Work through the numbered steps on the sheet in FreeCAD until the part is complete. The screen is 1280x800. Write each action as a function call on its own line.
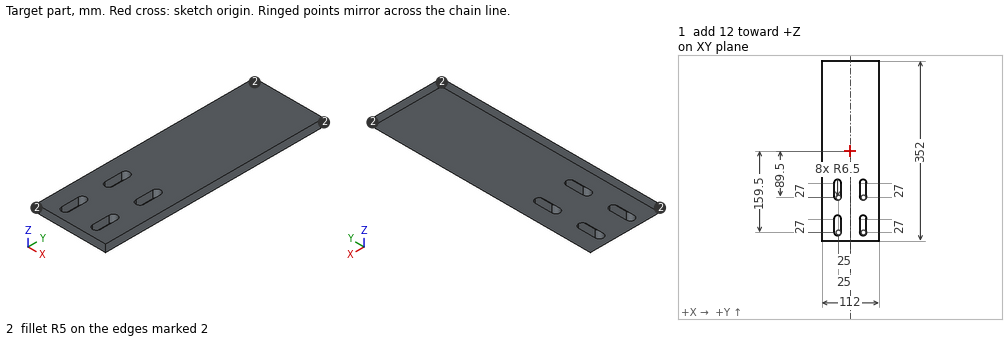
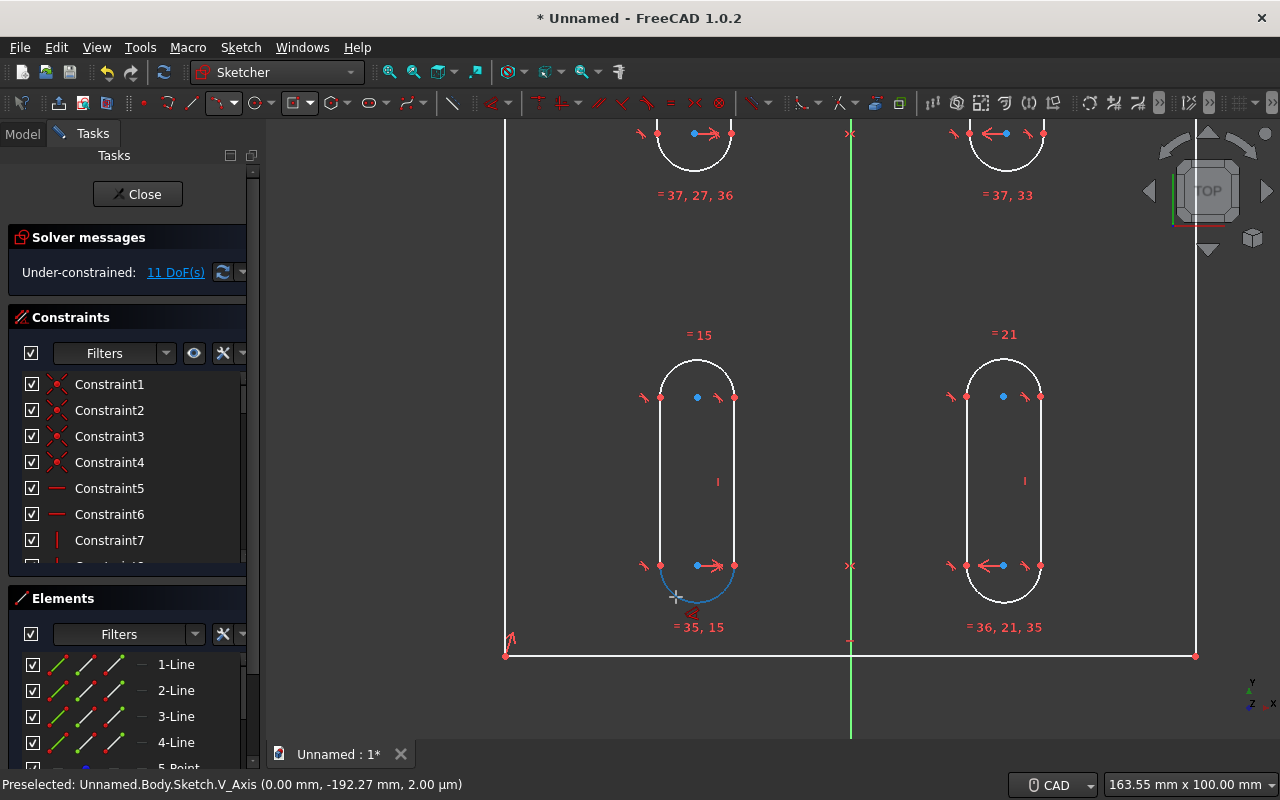
click(675, 596)
click(656, 622)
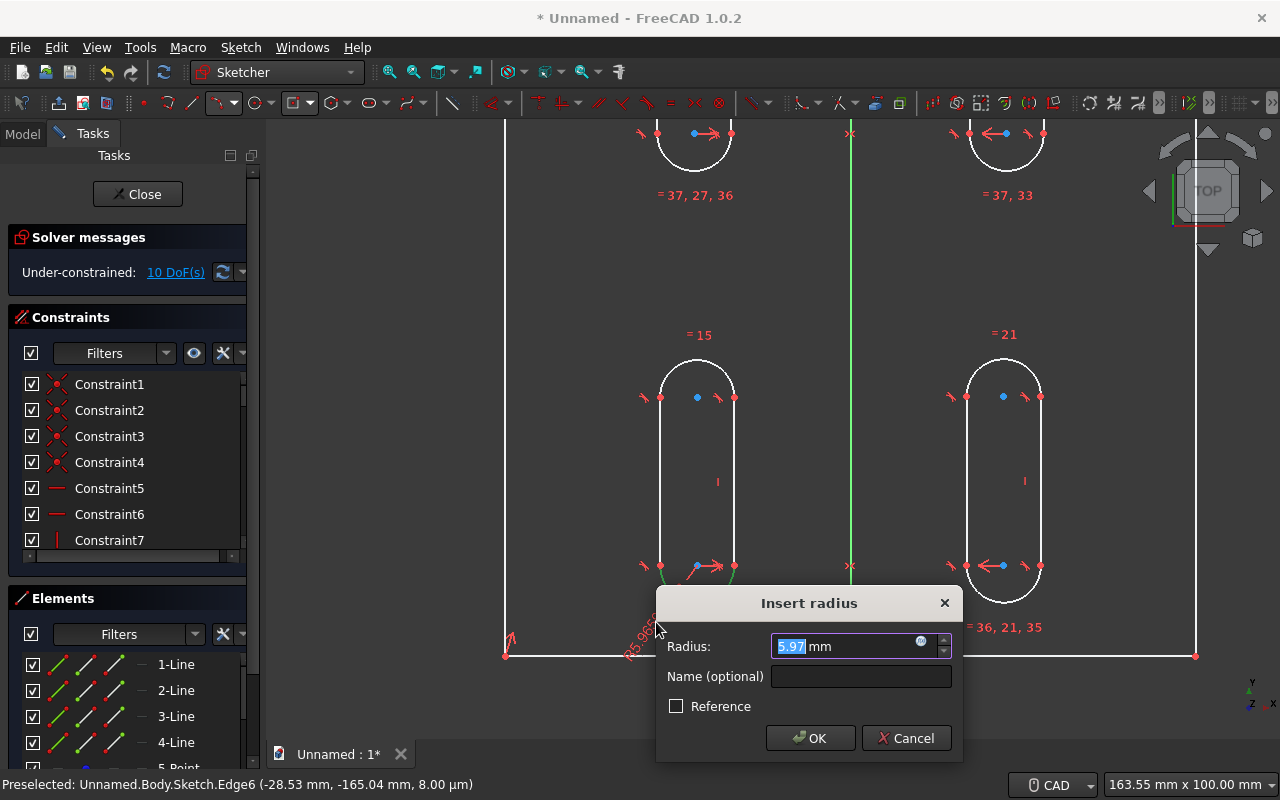
text(6.5)
key(Return)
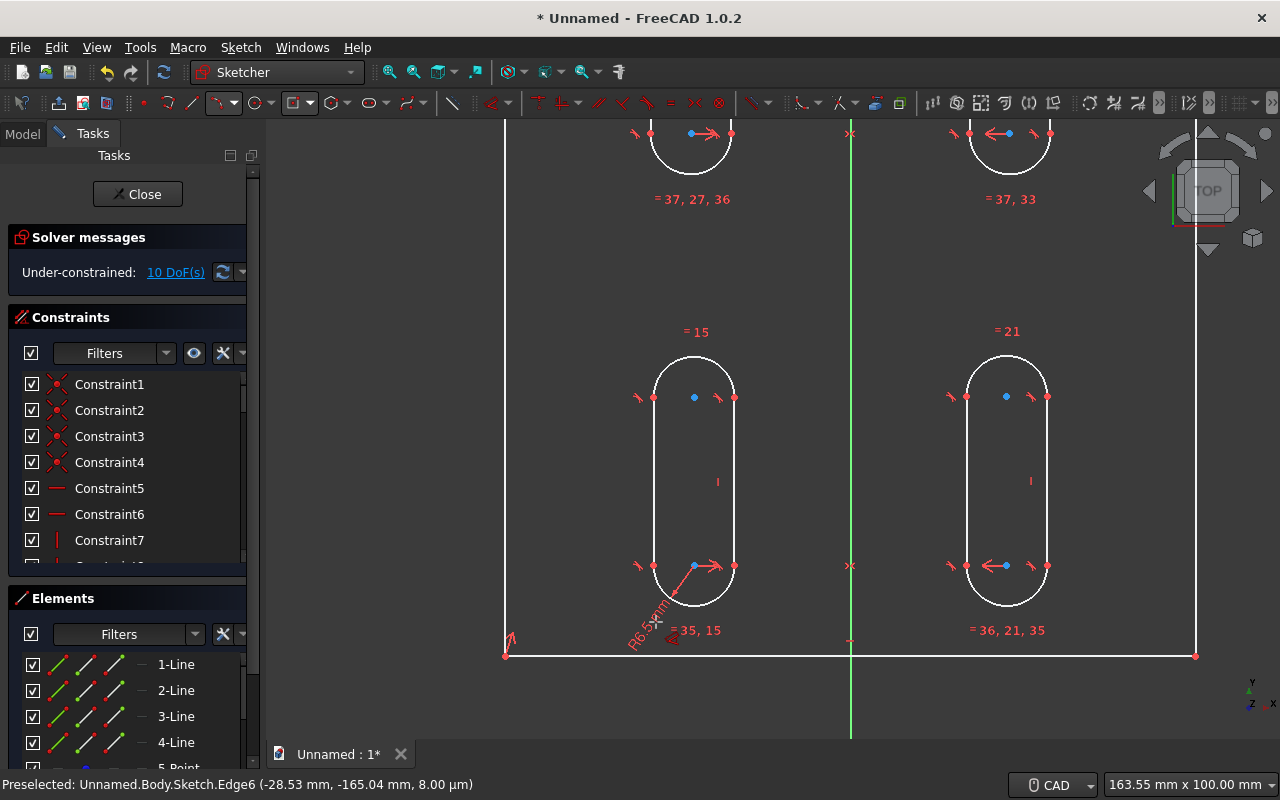
scroll(676, 599, down, 9)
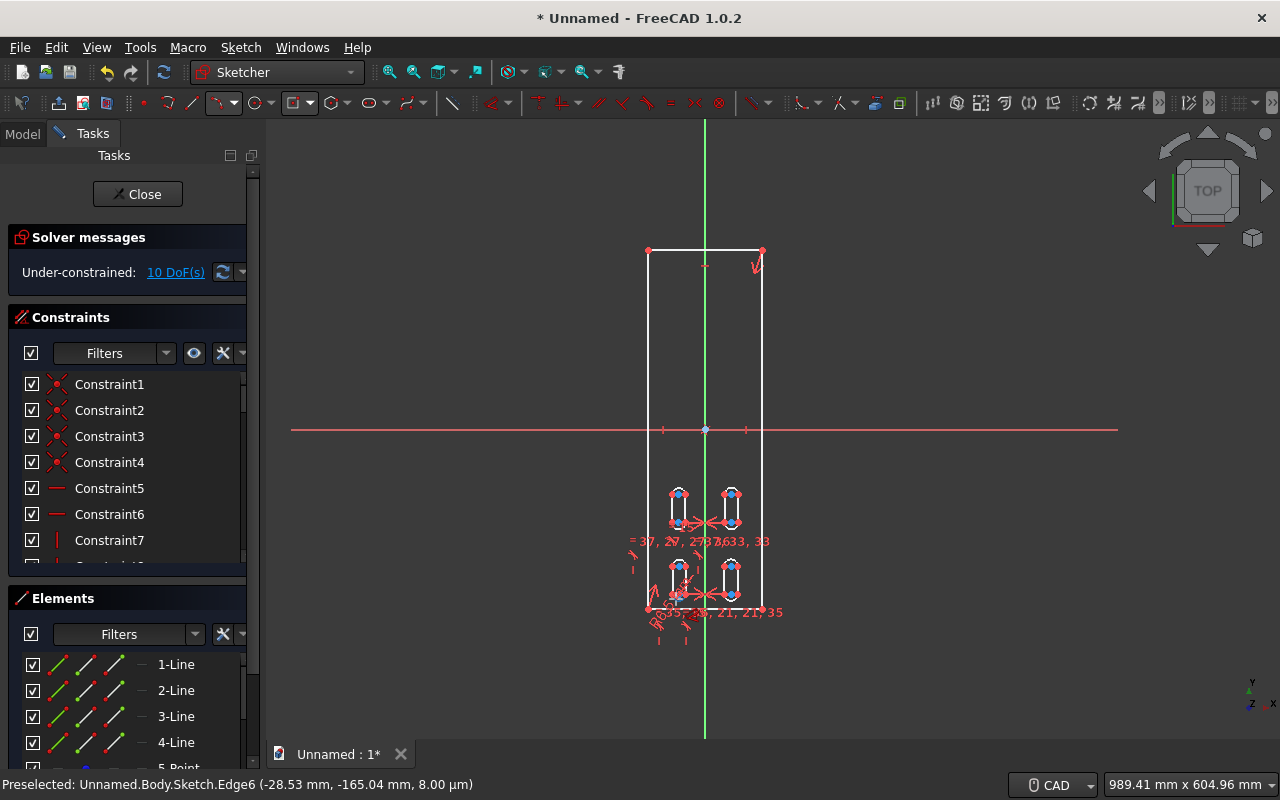
scroll(673, 586, up, 3)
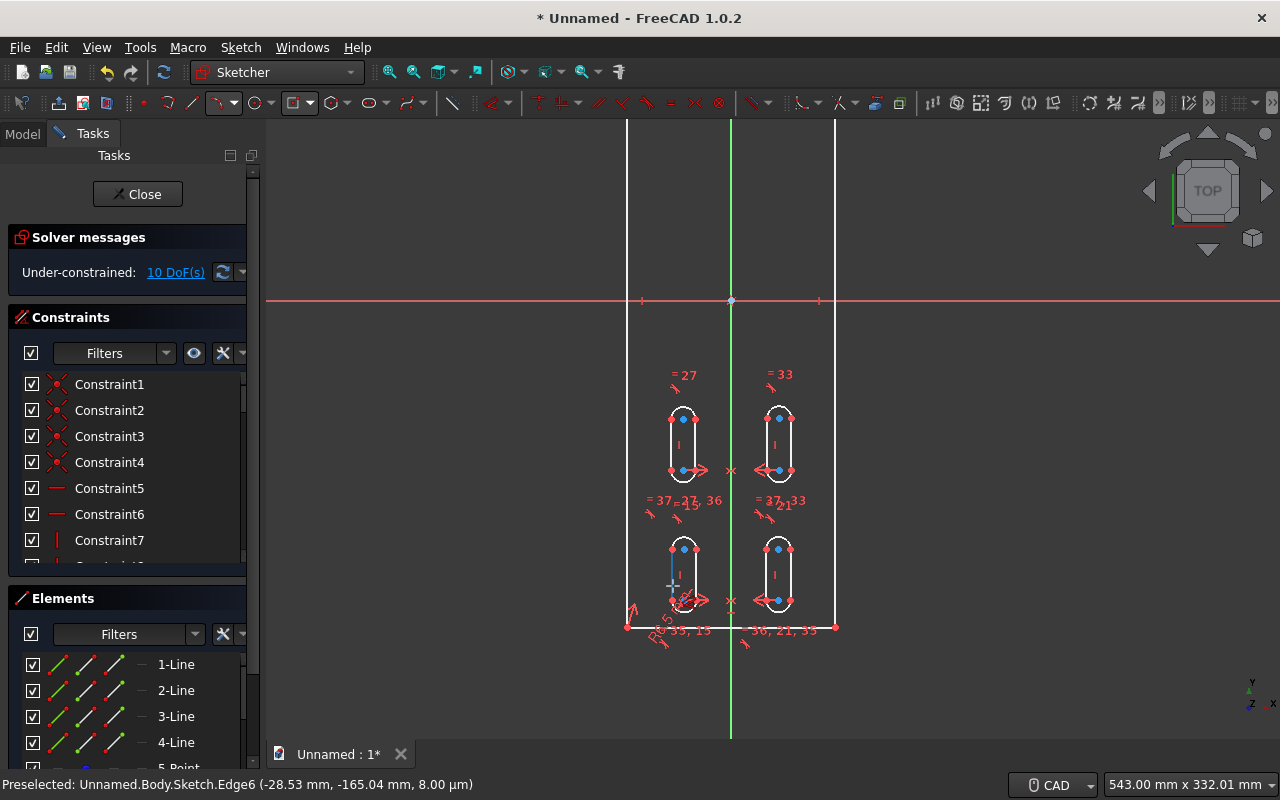
click(672, 585)
click(614, 575)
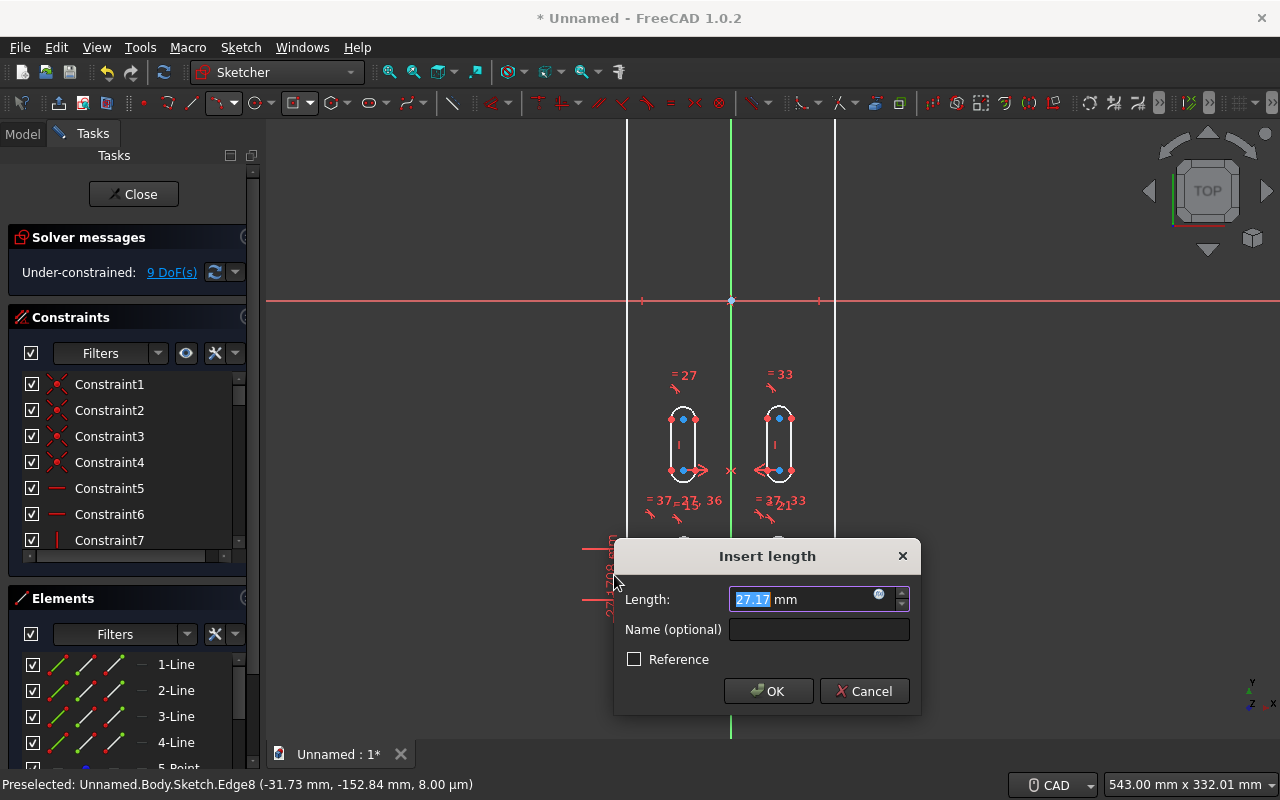
text(27)
key(Return)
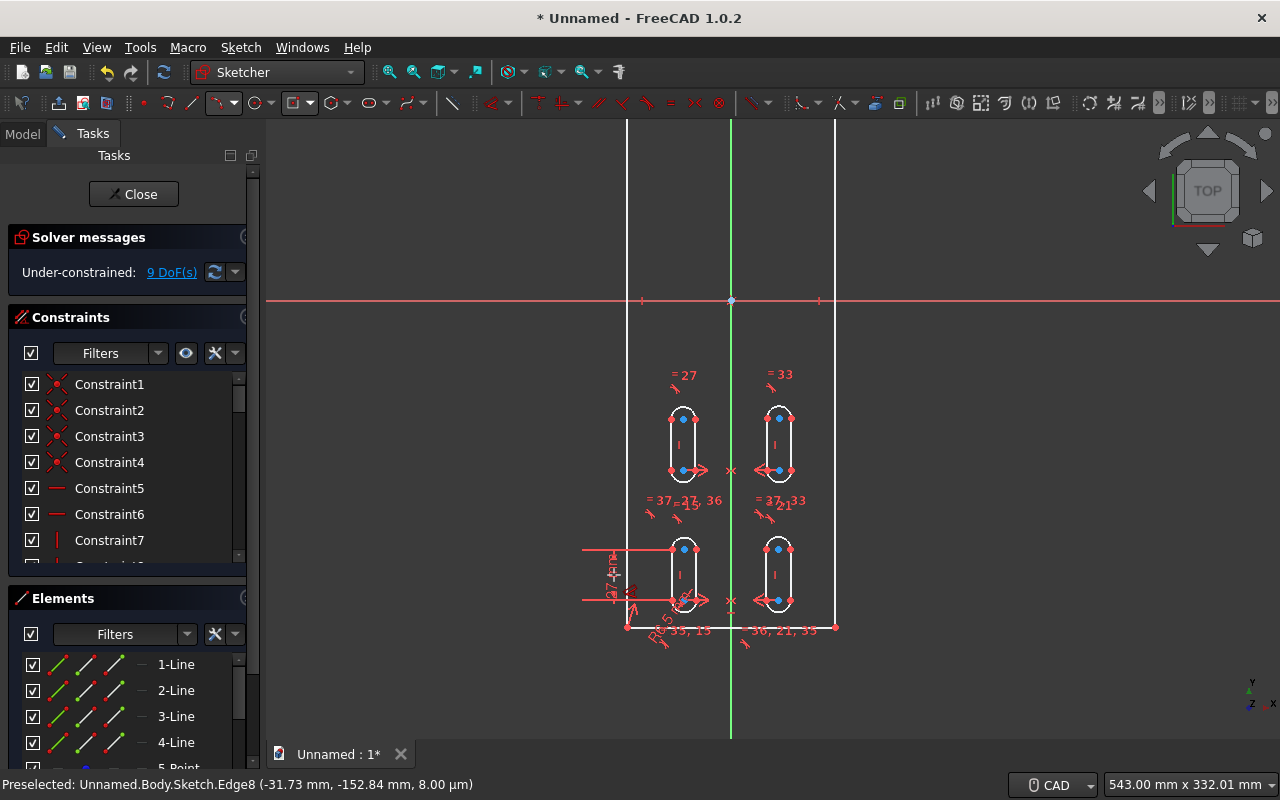
click(766, 585)
click(872, 575)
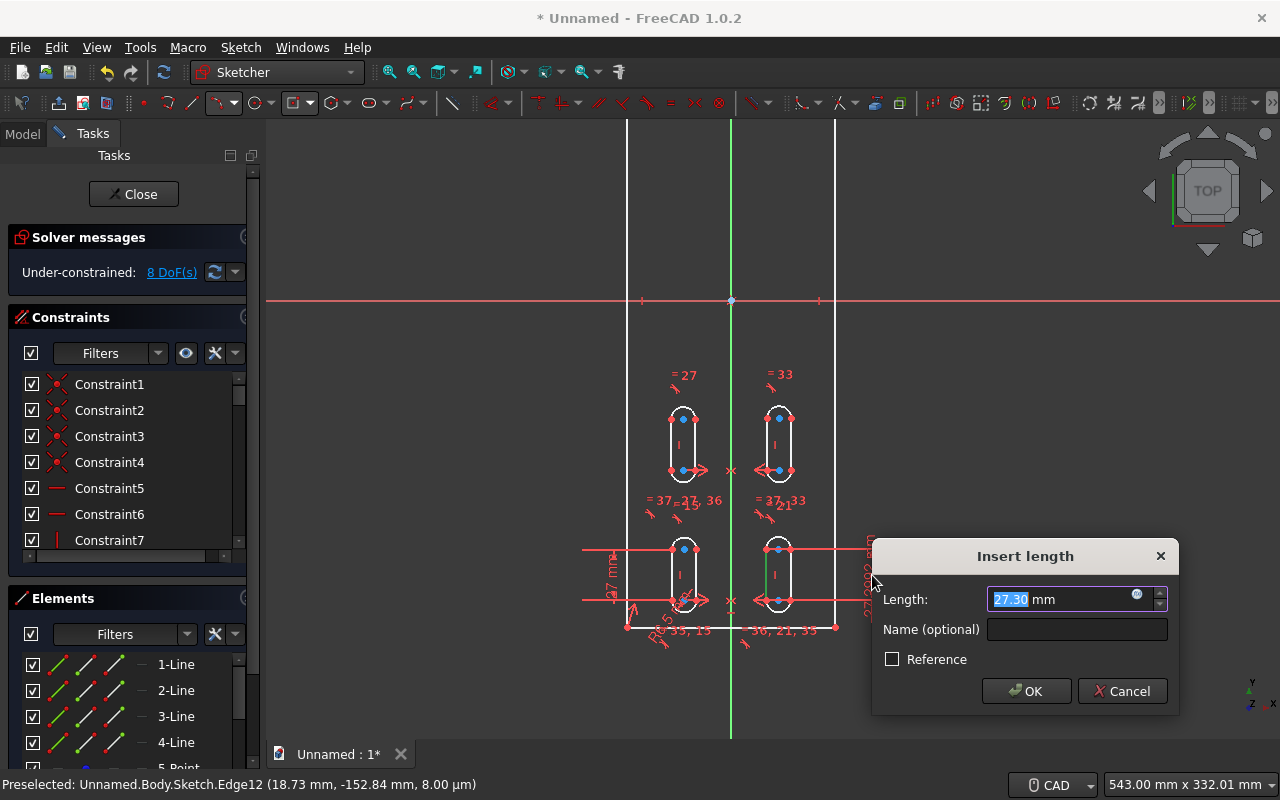
text(27)
key(Return)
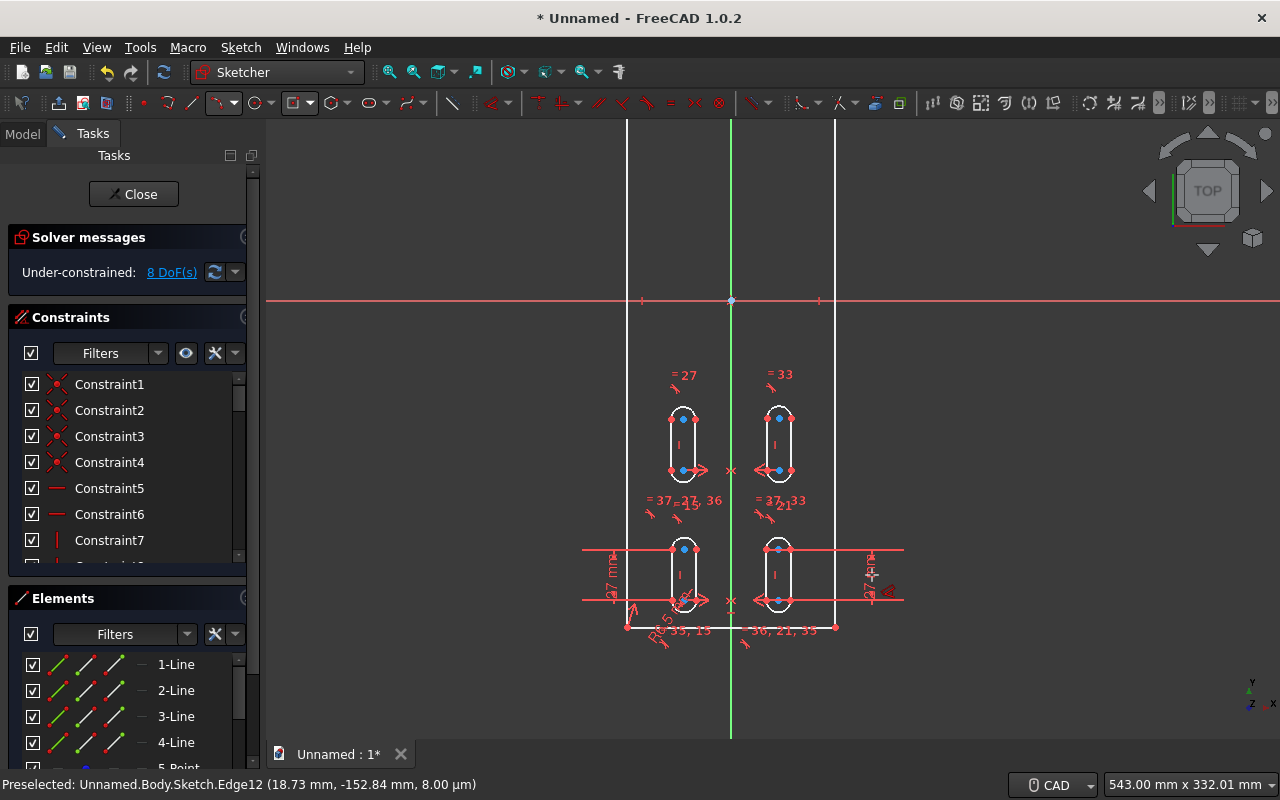
click(671, 455)
click(613, 445)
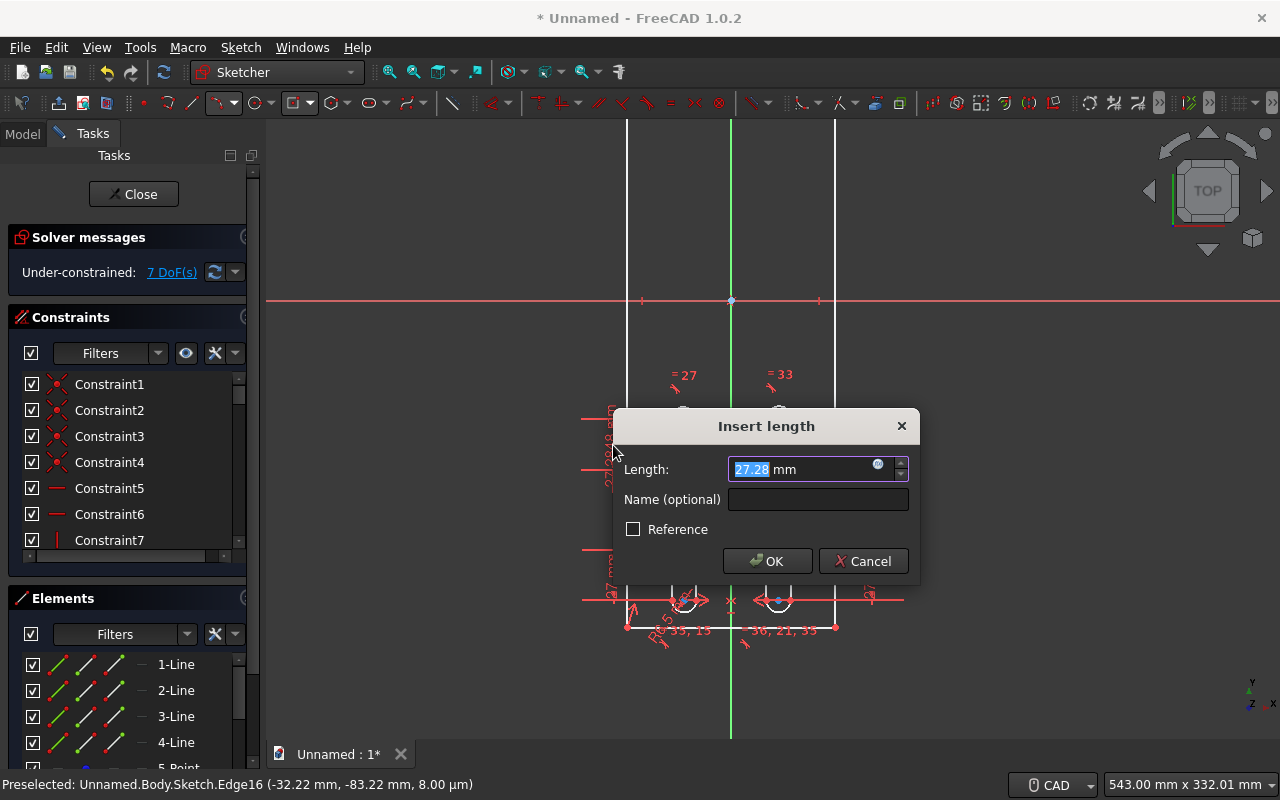
text(27)
key(Return)